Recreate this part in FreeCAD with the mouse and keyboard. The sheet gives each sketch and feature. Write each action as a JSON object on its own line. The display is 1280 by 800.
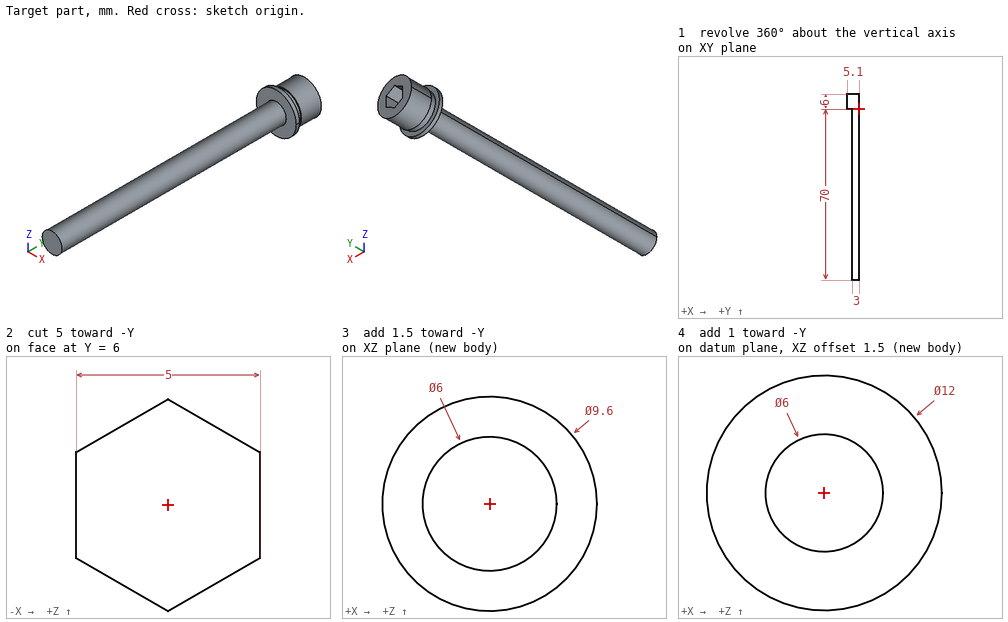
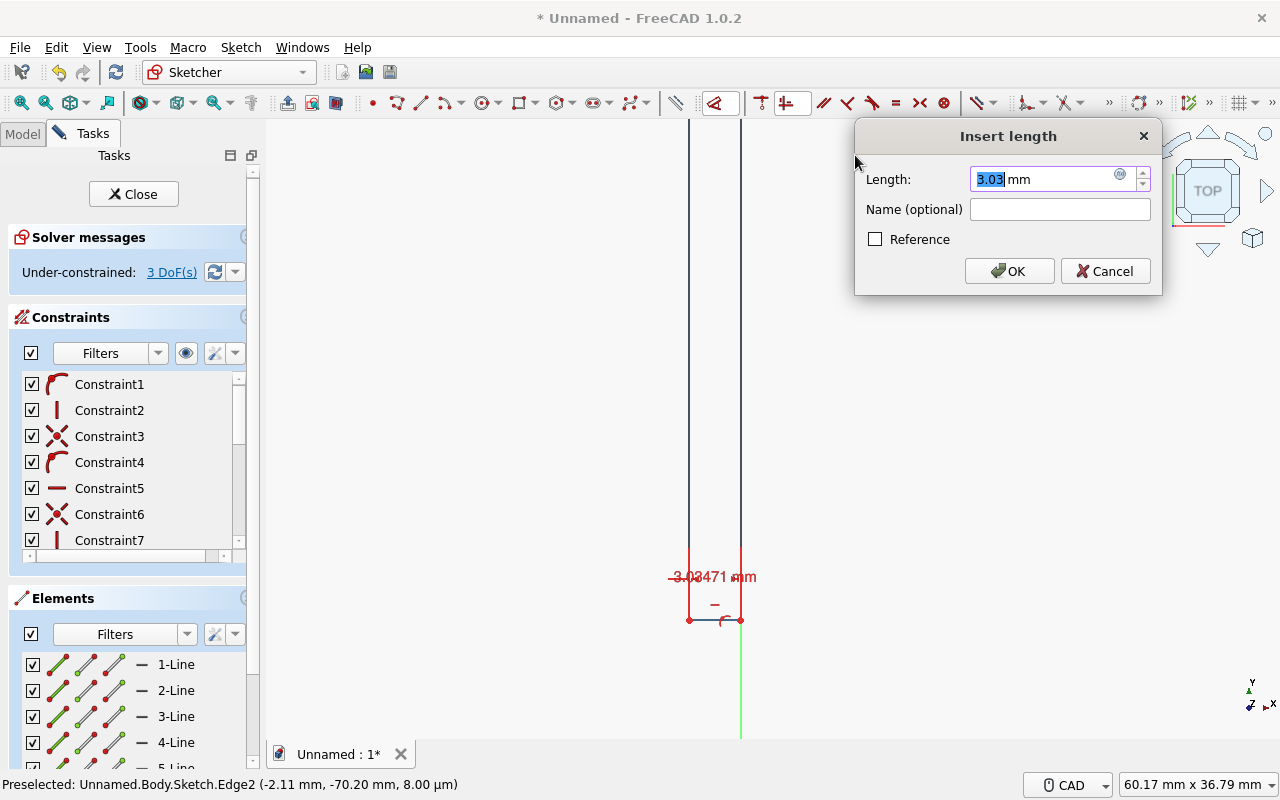
{"action": "type", "text": "3"}
{"action": "key", "text": "Return"}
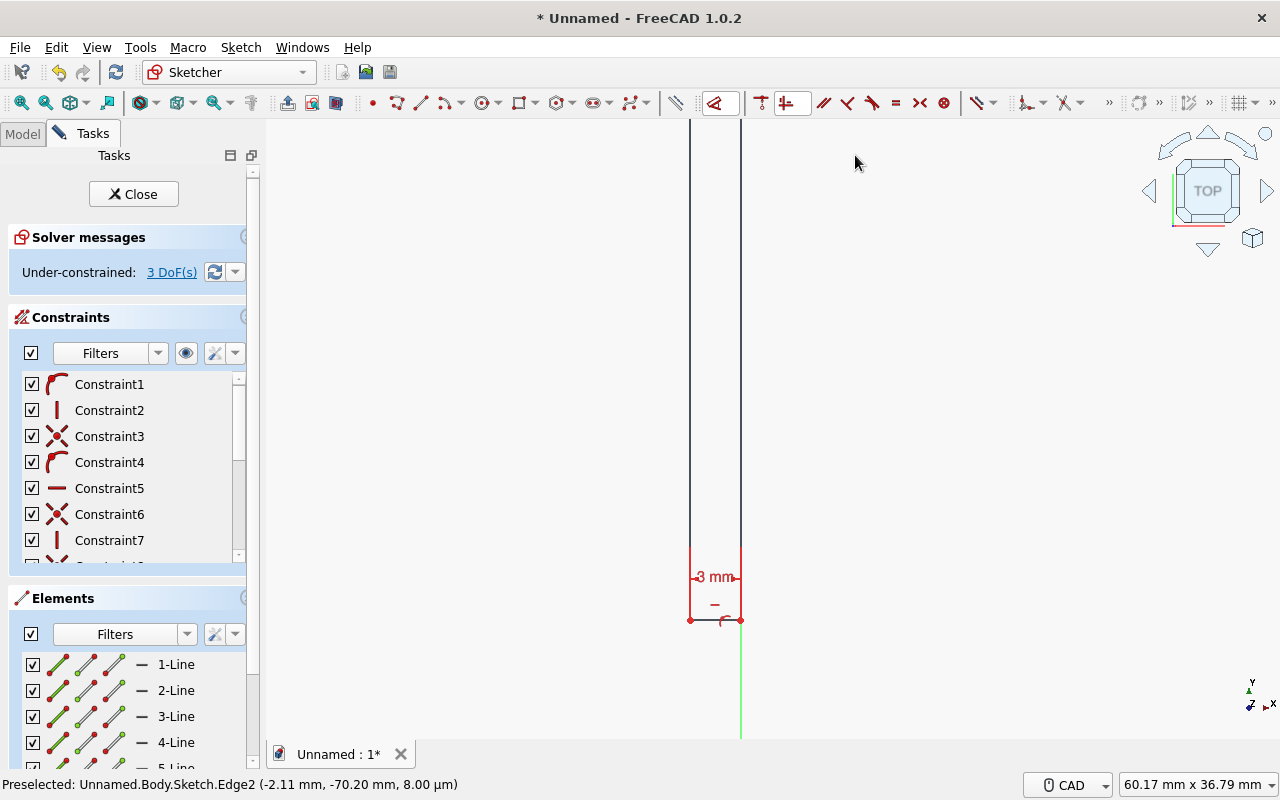
{"action": "scroll", "coordinate": [707, 624], "scroll_direction": "down", "scroll_amount": 6}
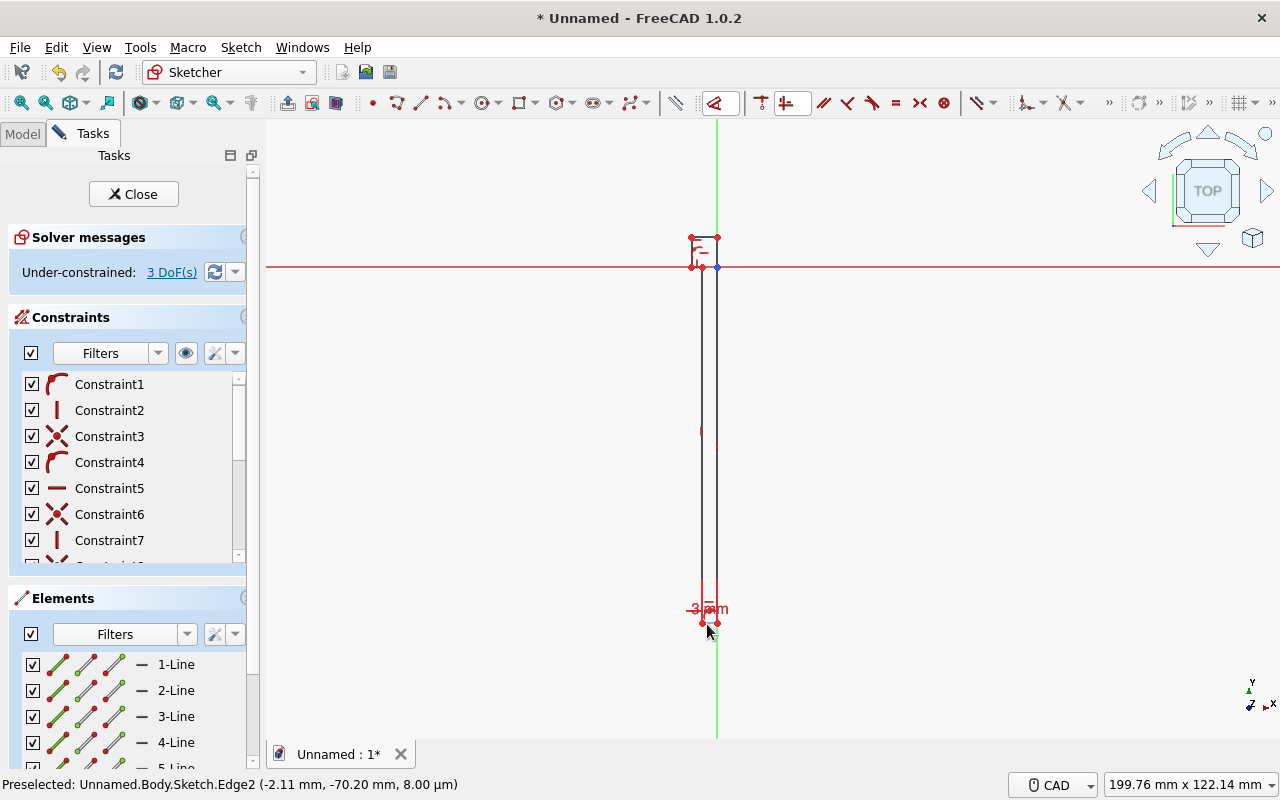
{"action": "scroll", "coordinate": [692, 246], "scroll_direction": "up", "scroll_amount": 3}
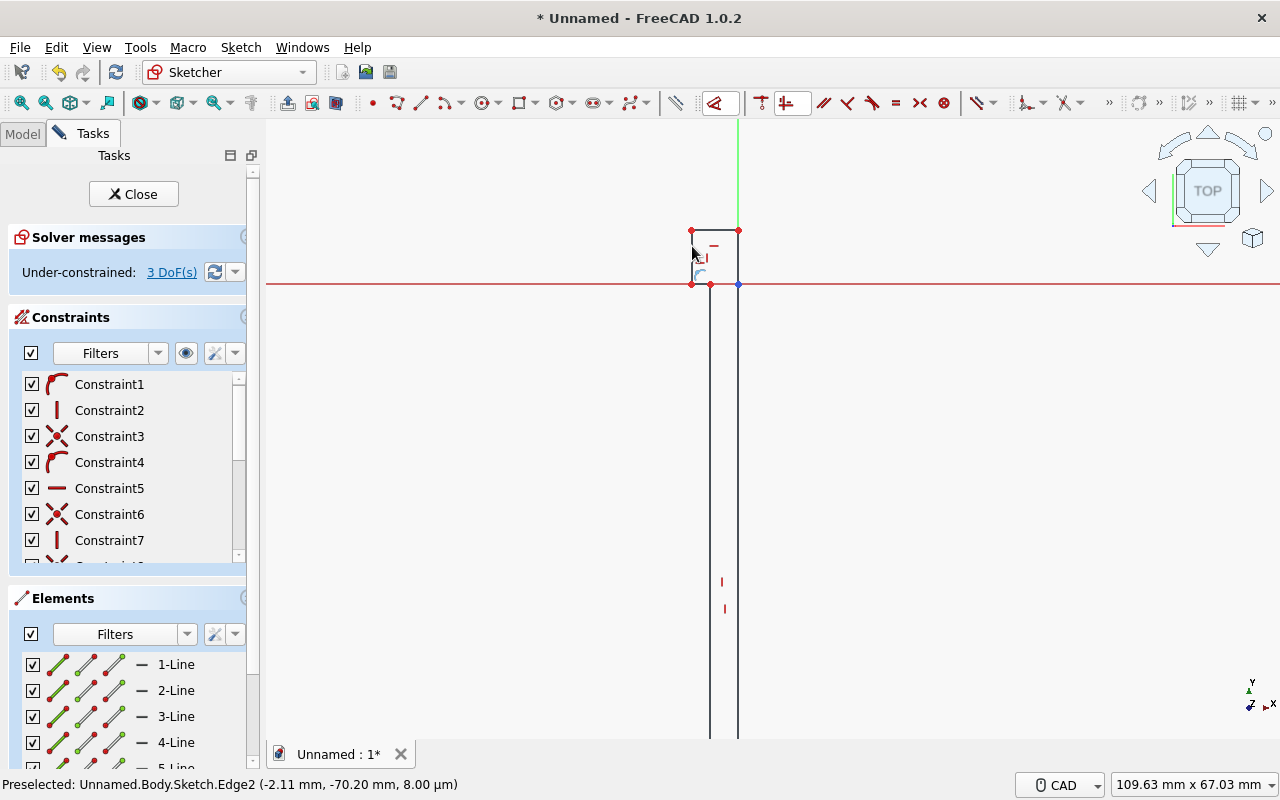
{"action": "left_click", "coordinate": [692, 247]}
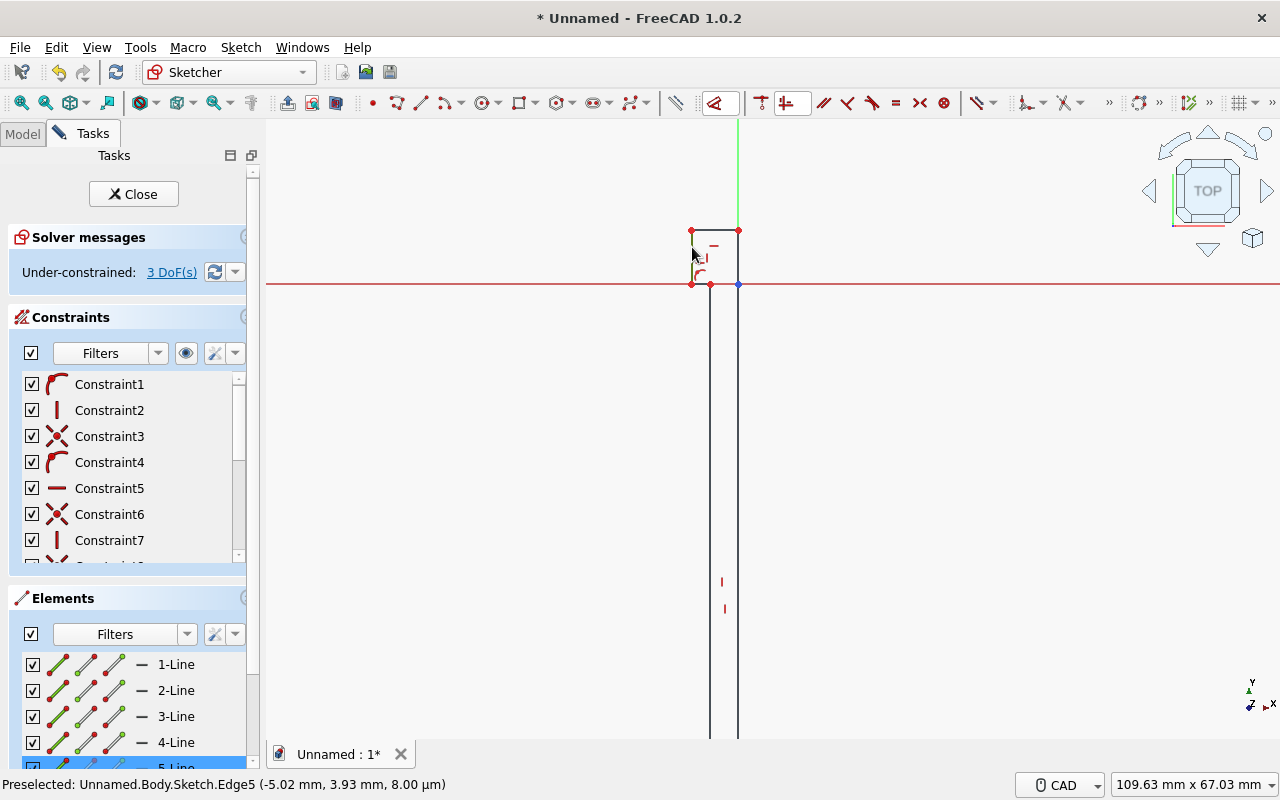
{"action": "key", "text": "i"}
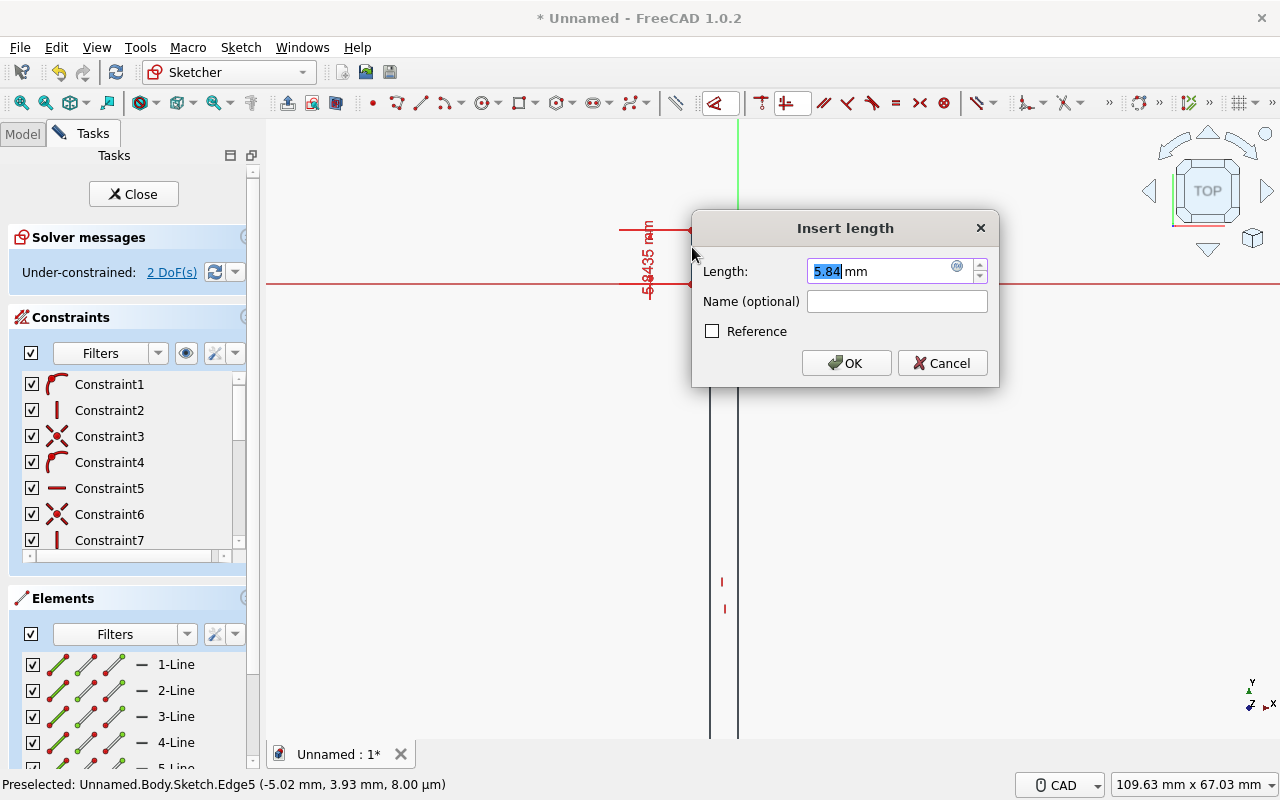
{"action": "type", "text": "6"}
{"action": "key", "text": "Return"}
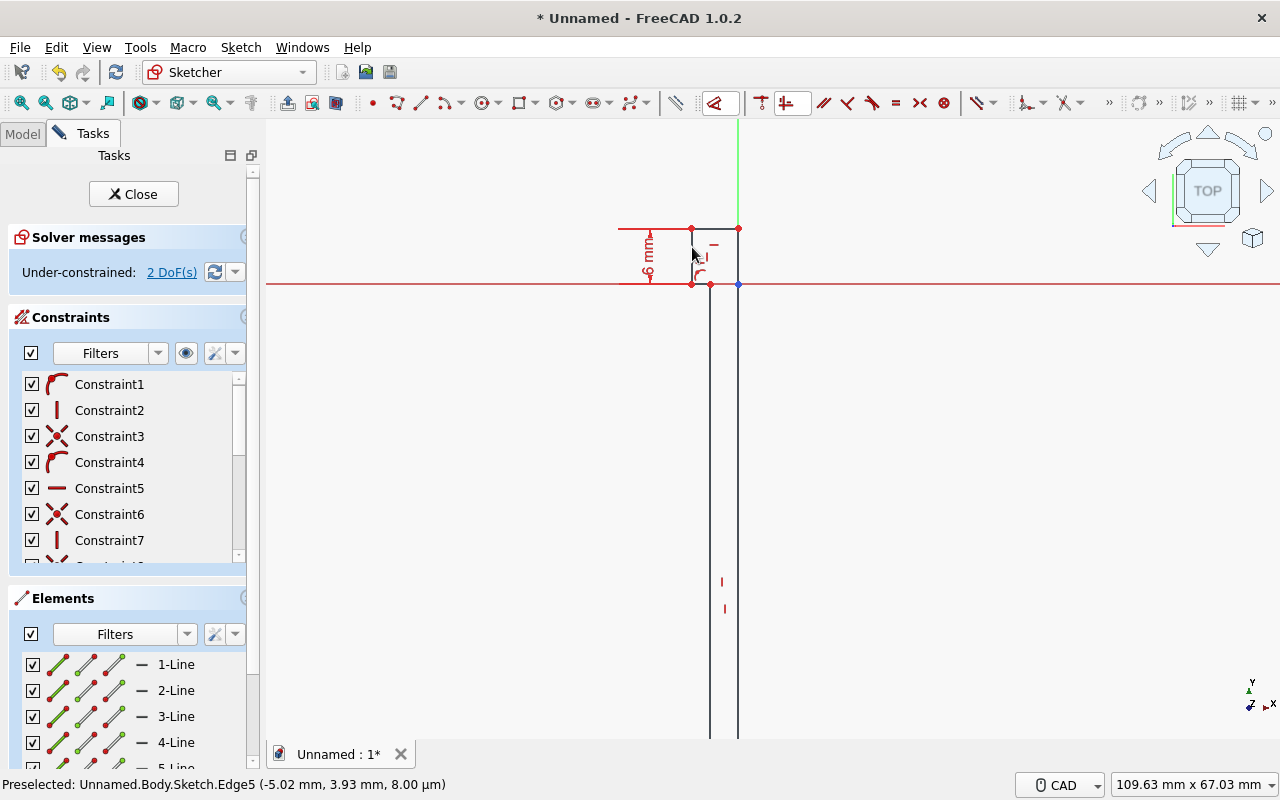
{"action": "left_click", "coordinate": [710, 479]}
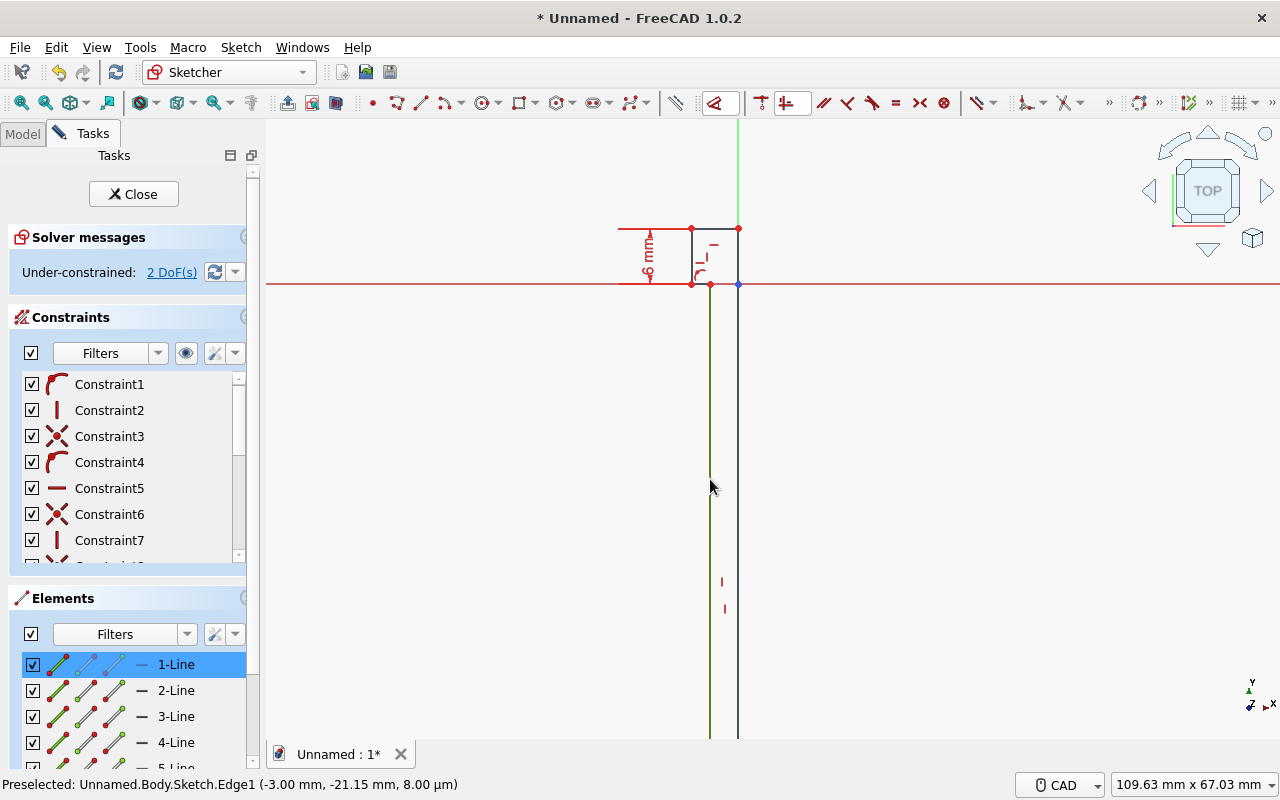
{"action": "key", "text": "i"}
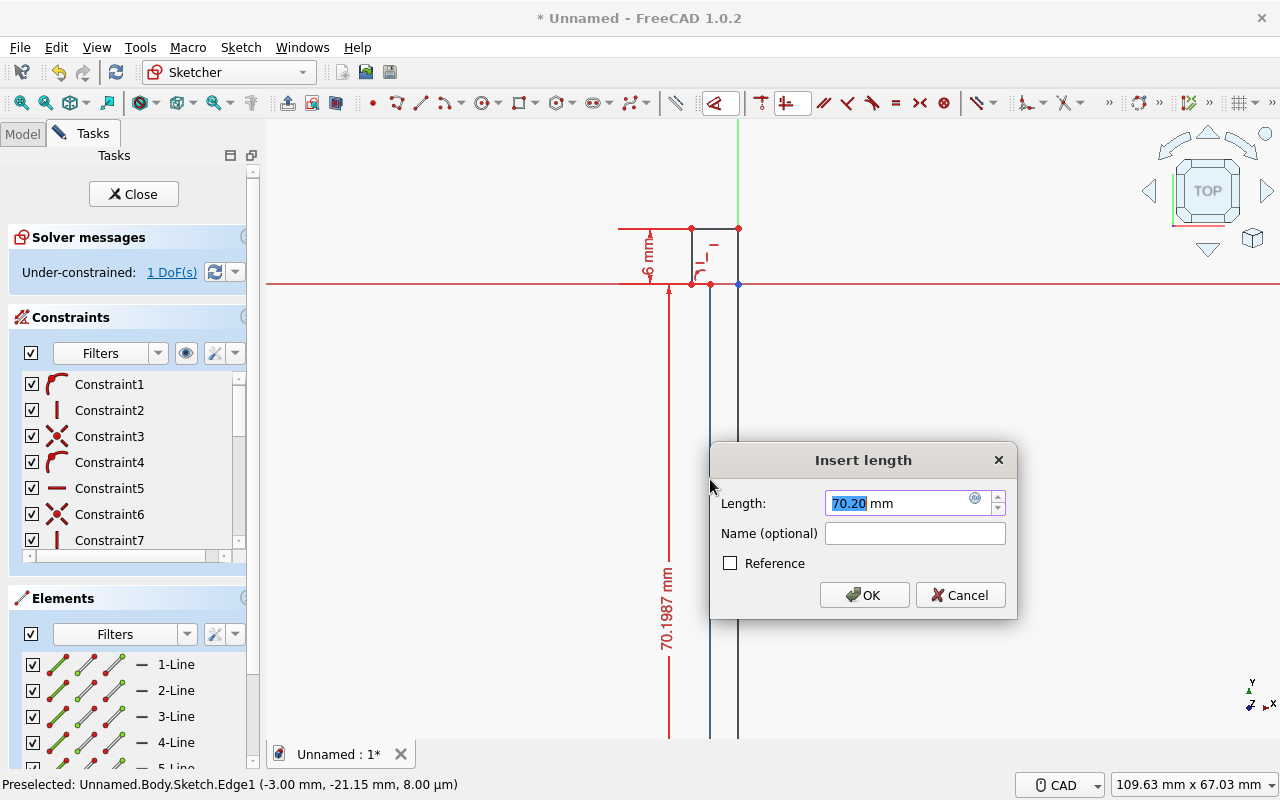
{"action": "type", "text": "70"}
{"action": "key", "text": "Return"}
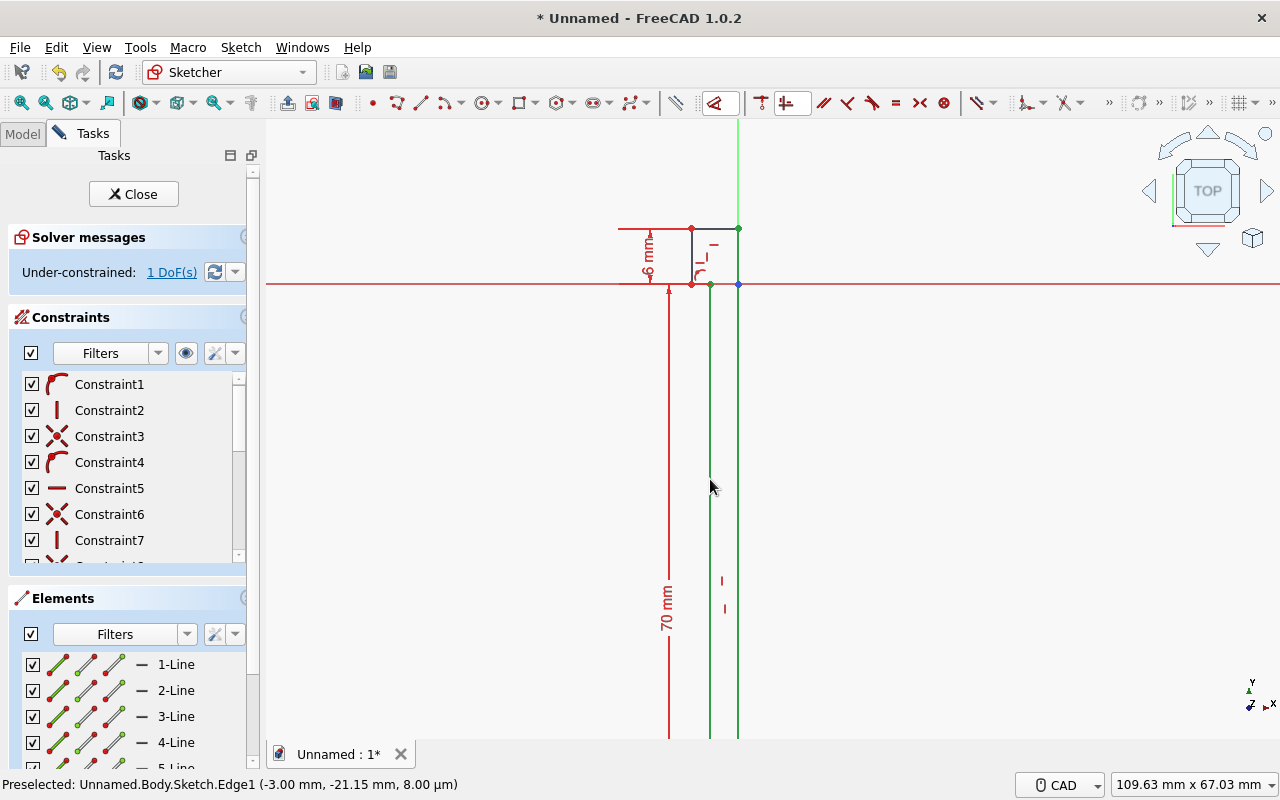
{"action": "left_click", "coordinate": [724, 229]}